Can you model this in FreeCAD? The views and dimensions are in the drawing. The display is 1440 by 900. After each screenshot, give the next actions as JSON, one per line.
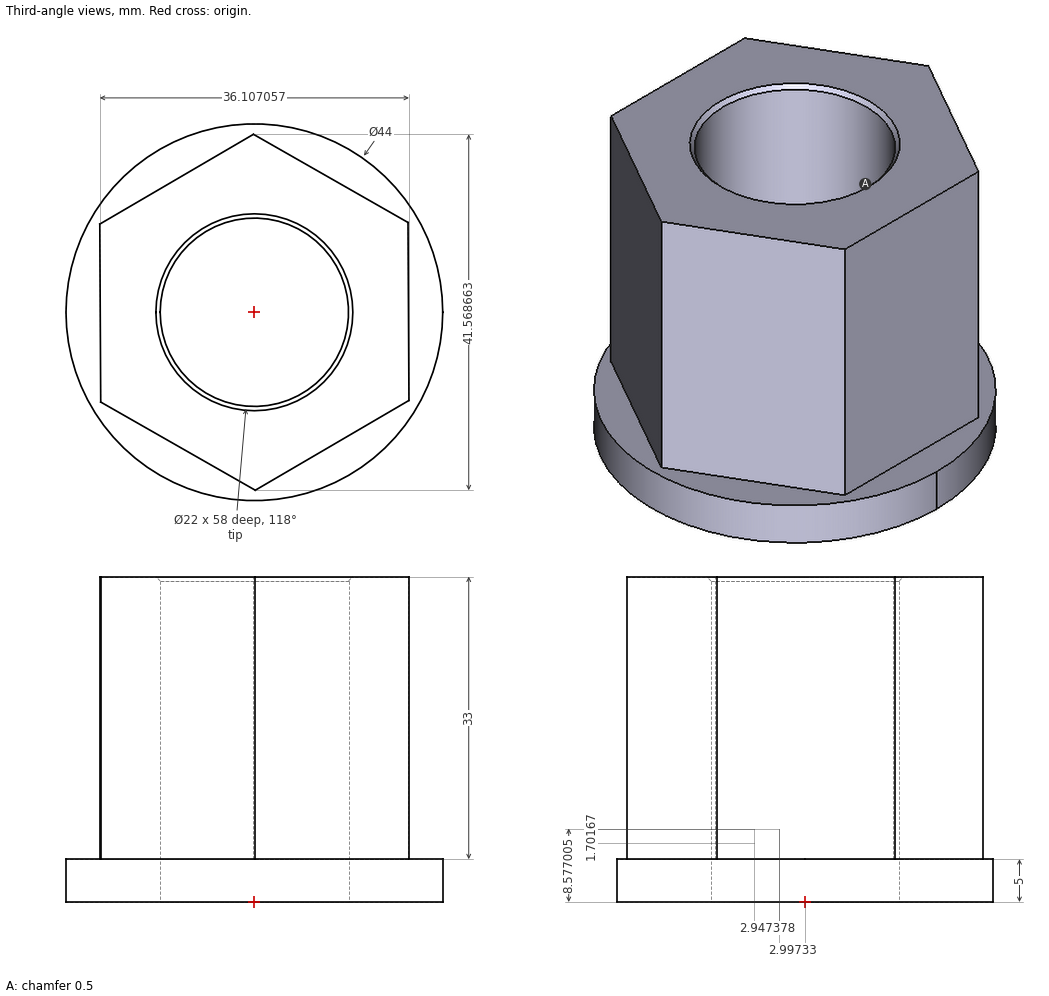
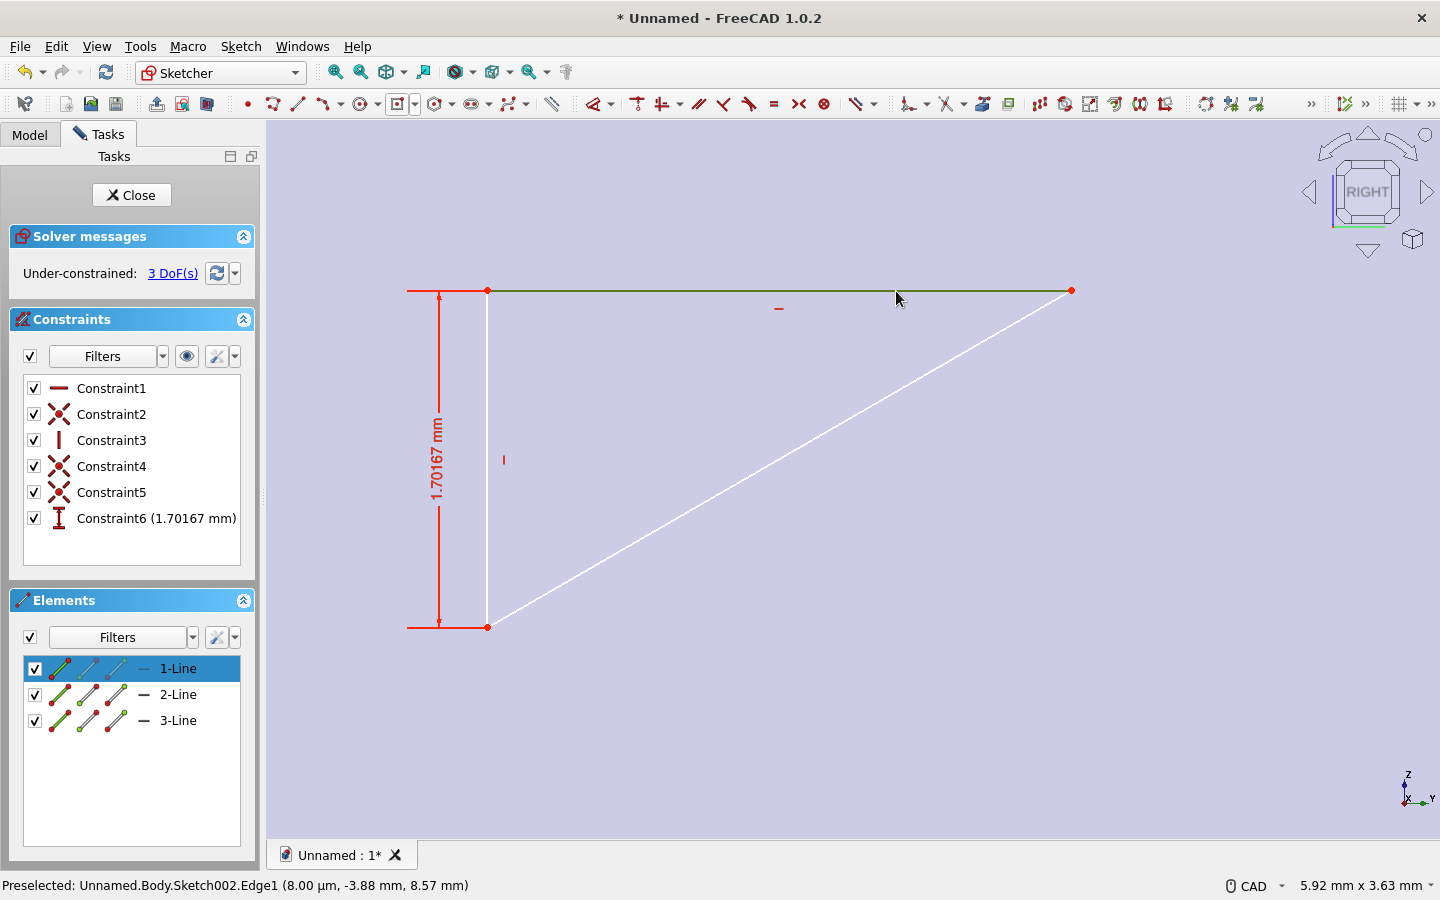
{"action": "key", "text": "l"}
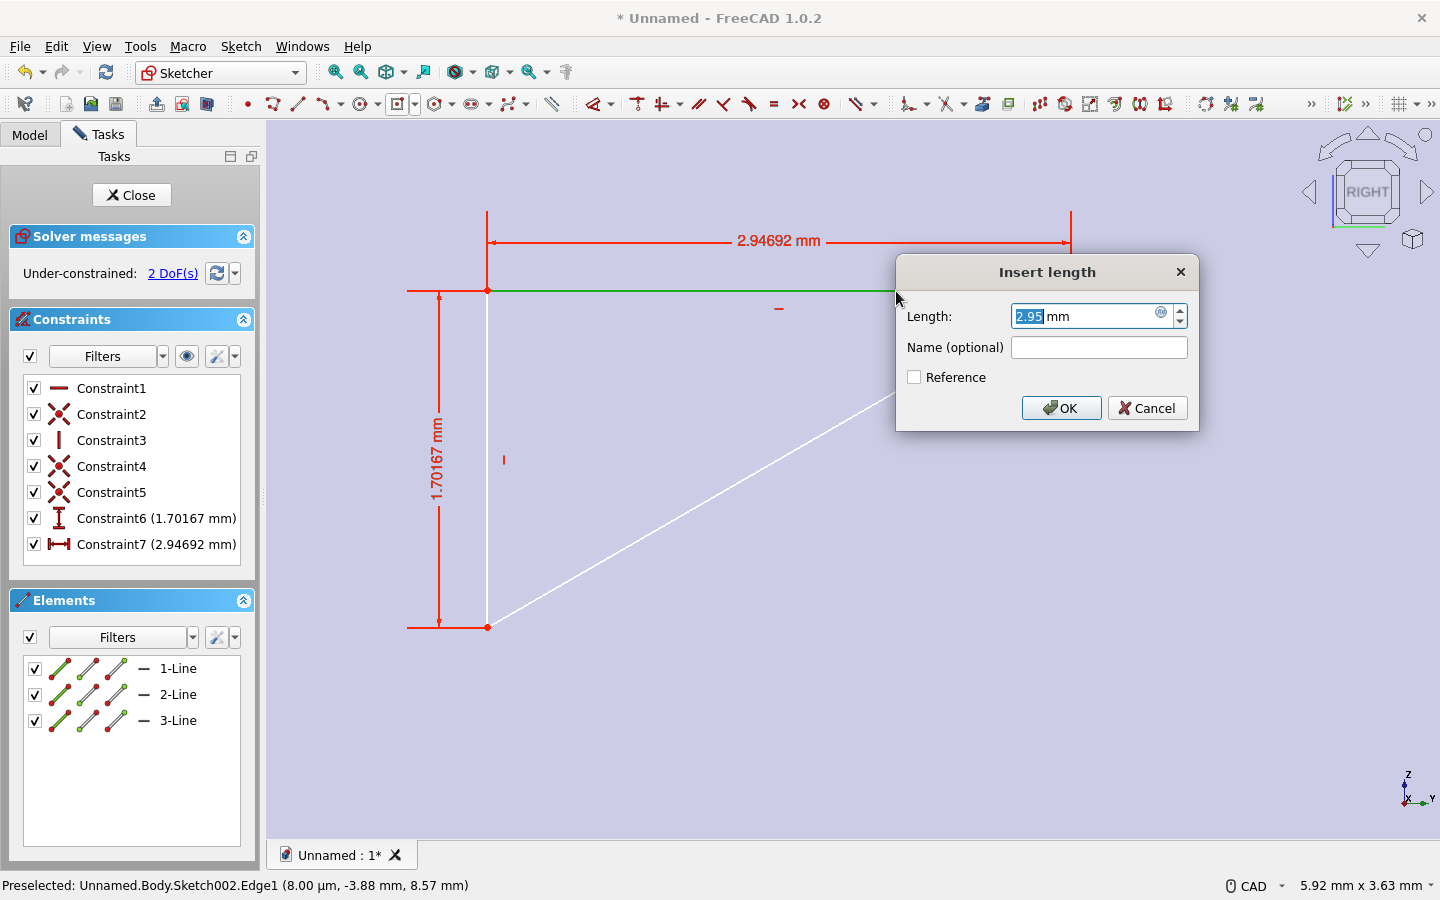
{"action": "type", "text": "2.947378"}
{"action": "key", "text": "Return"}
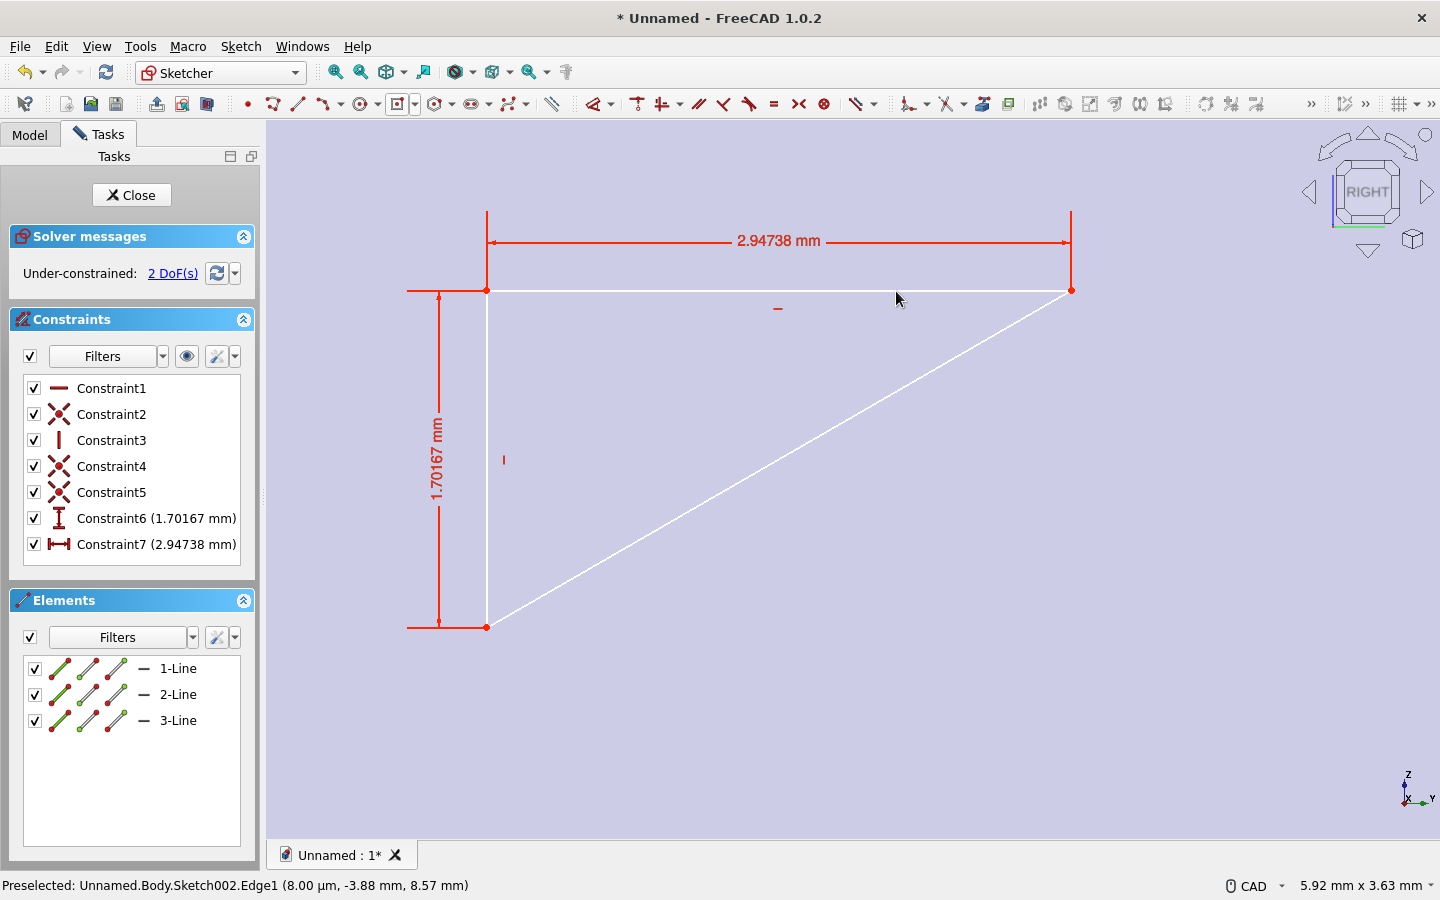
{"action": "left_click", "coordinate": [1071, 291]}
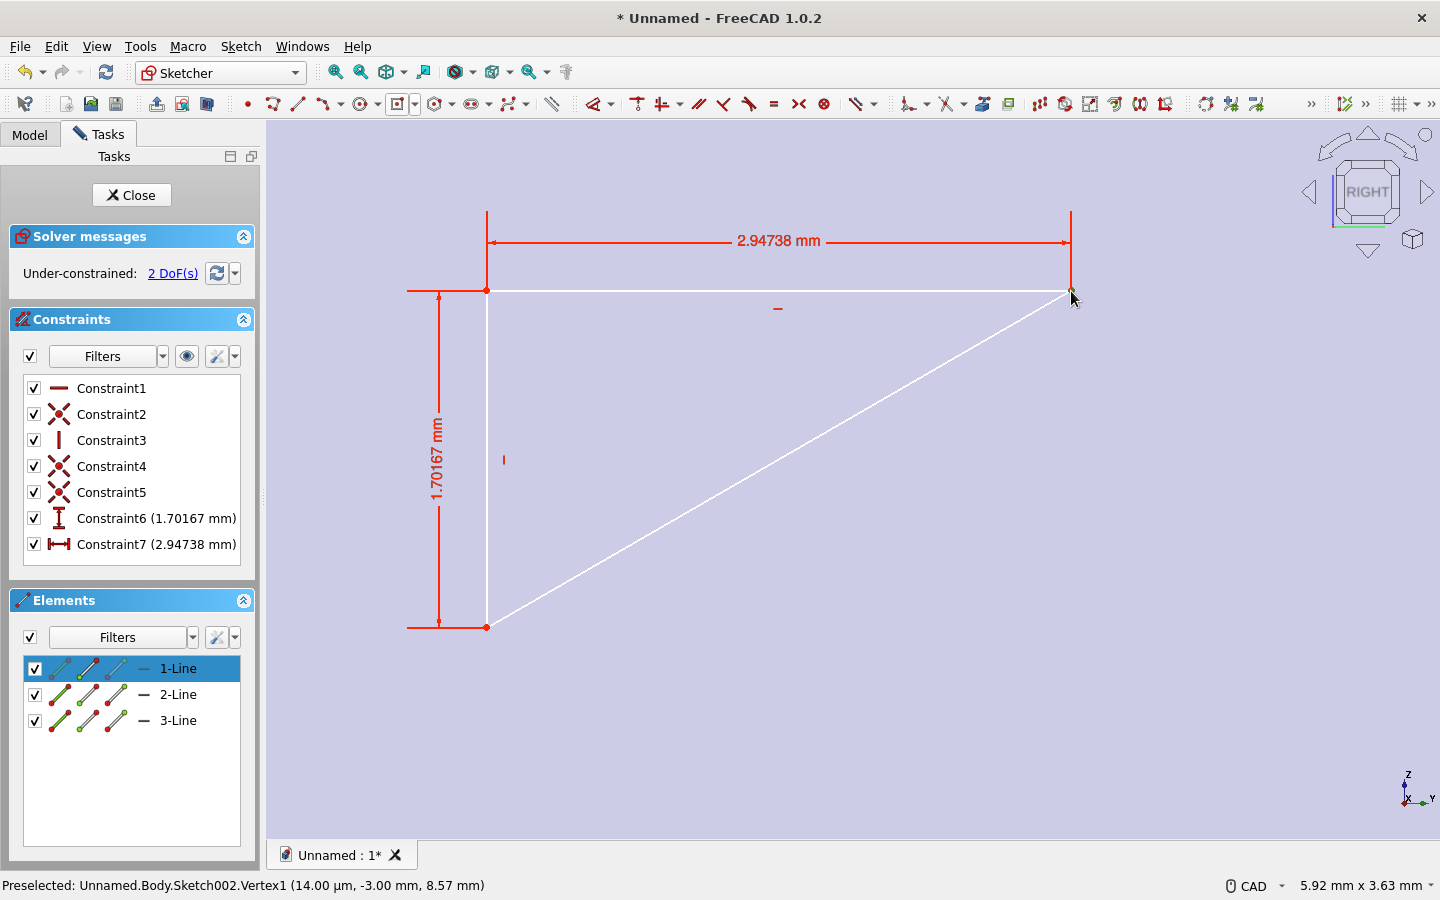
{"action": "key", "text": "l"}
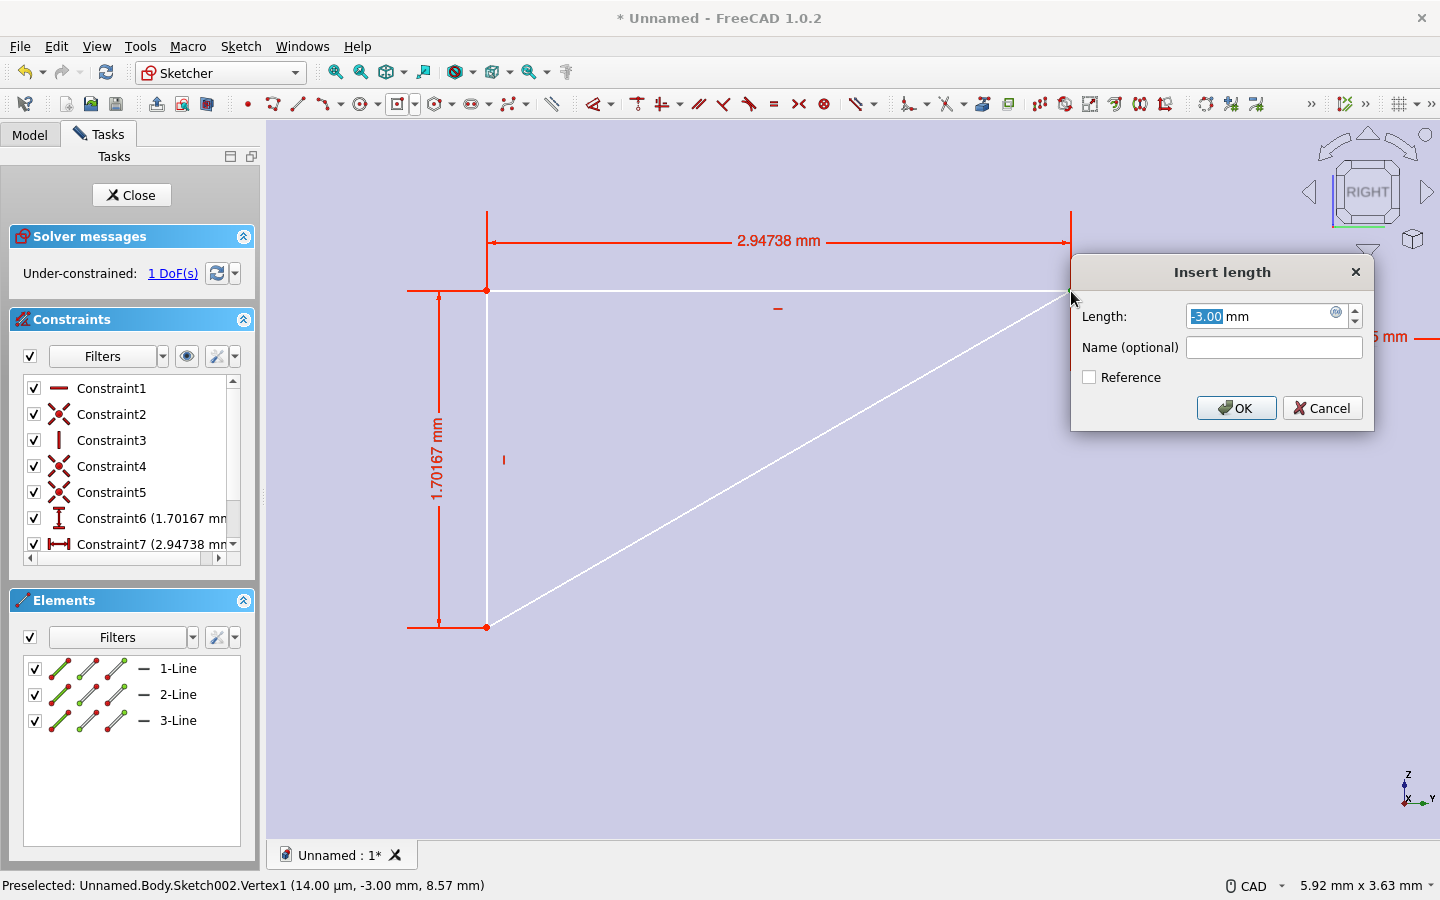
{"action": "type", "text": "-2.99733"}
{"action": "key", "text": "Return"}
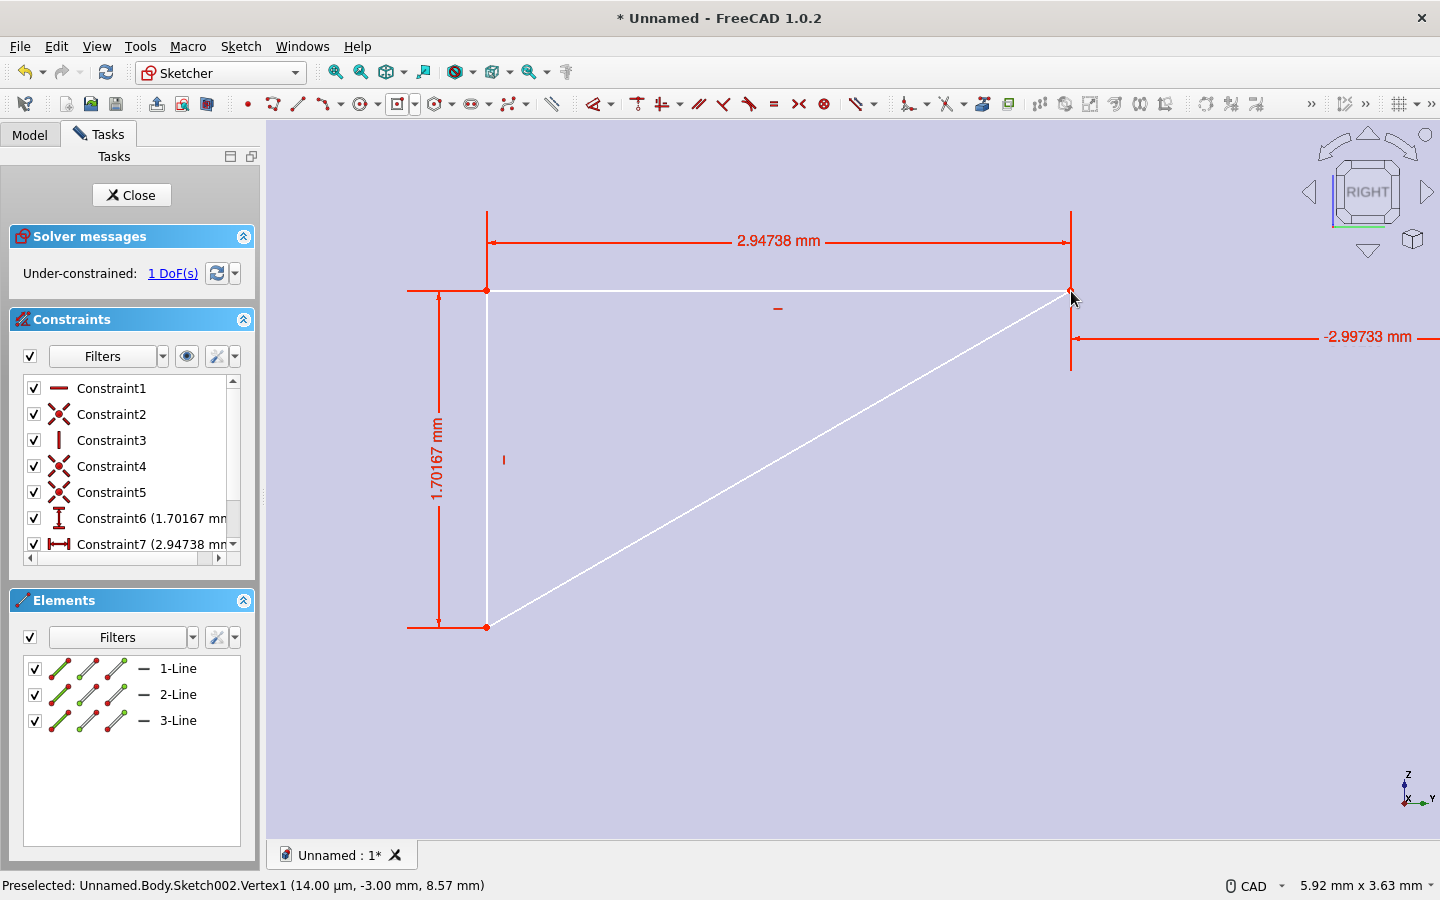
{"action": "left_click", "coordinate": [1071, 291]}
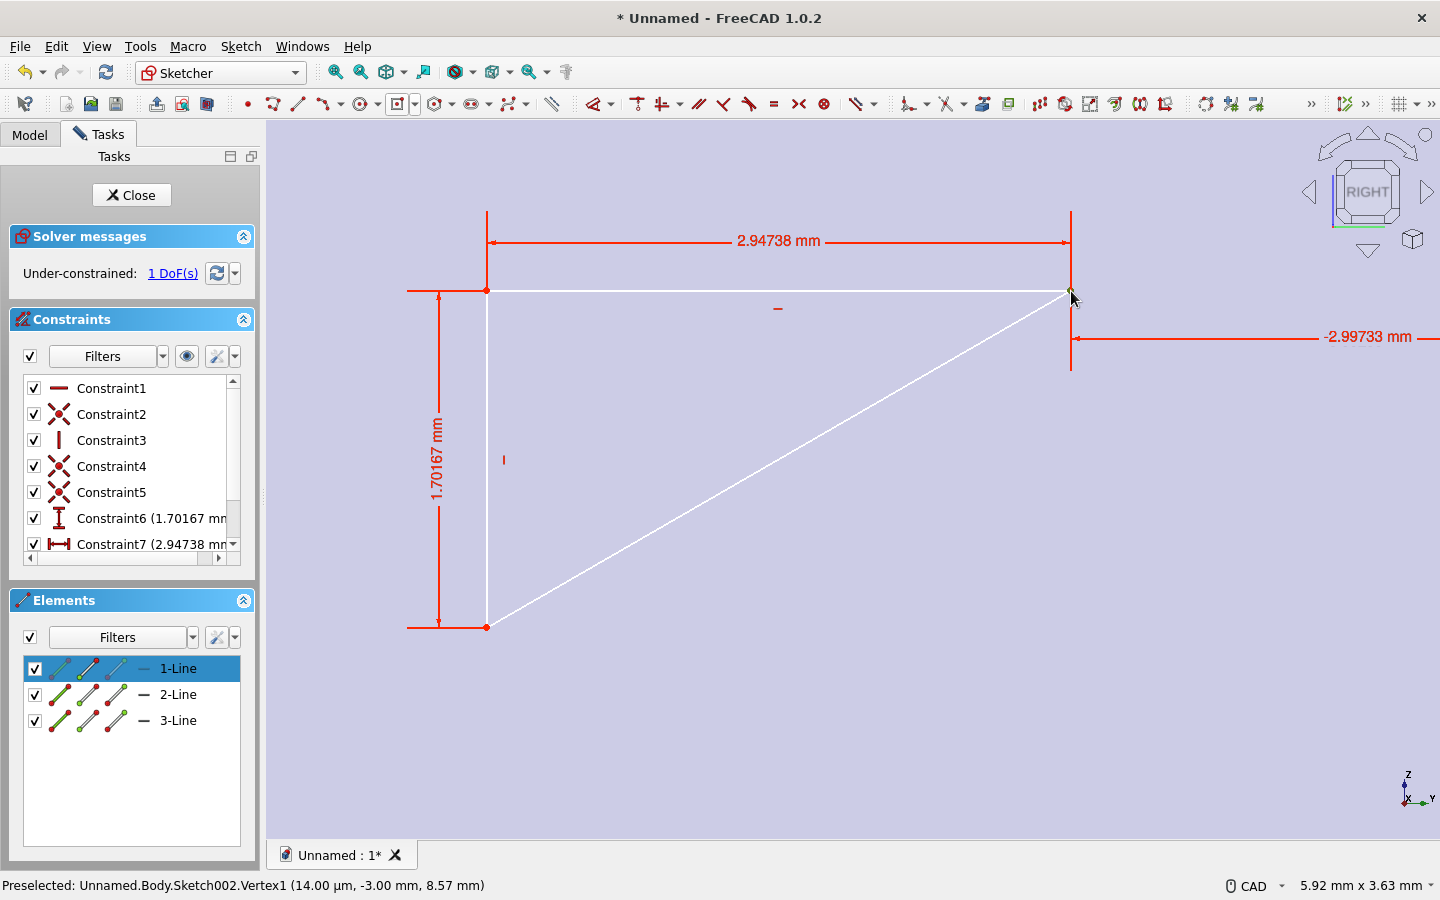
{"action": "key", "text": "i"}